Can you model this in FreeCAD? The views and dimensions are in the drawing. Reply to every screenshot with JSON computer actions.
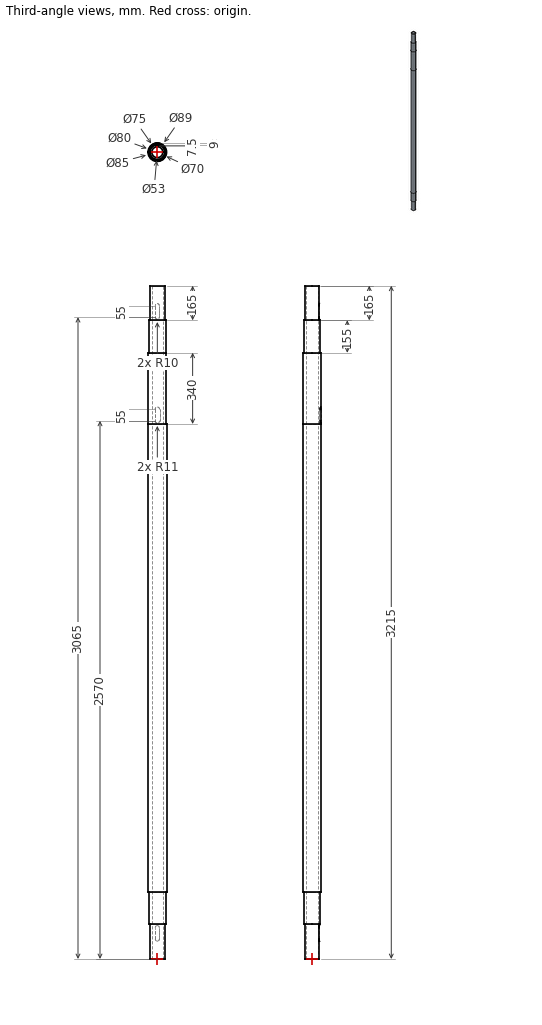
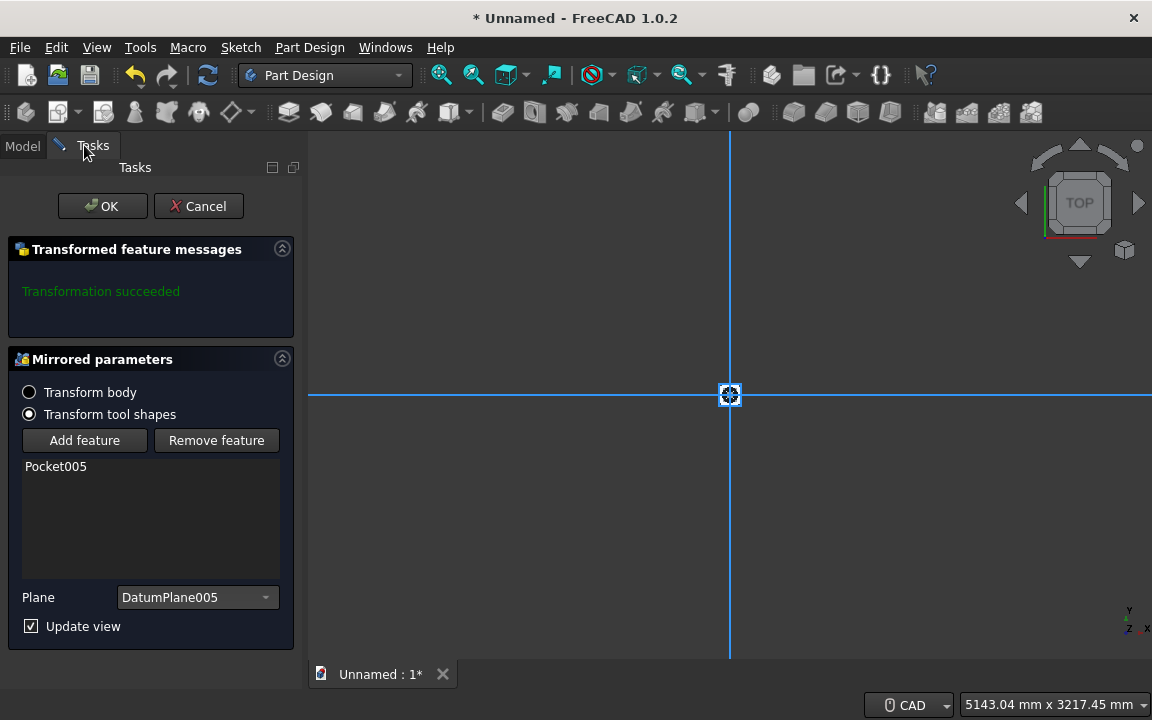
{"action": "left_click", "coordinate": [103, 206]}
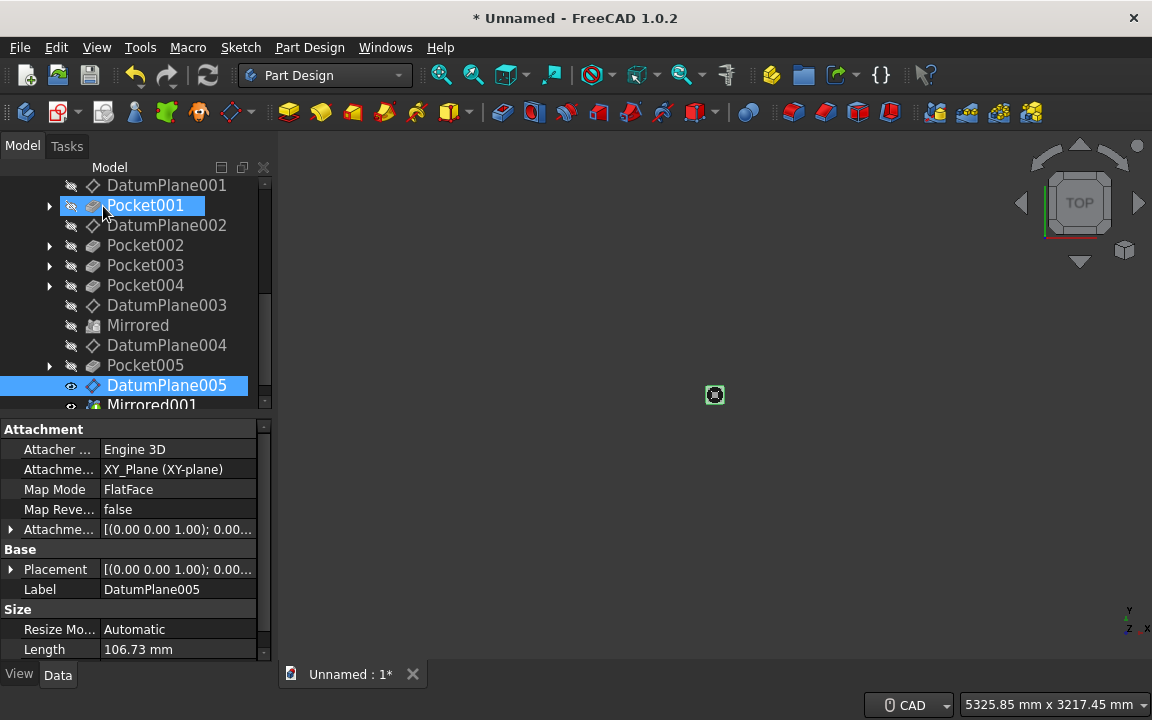
{"action": "left_click", "coordinate": [116, 386]}
{"action": "key", "text": "space"}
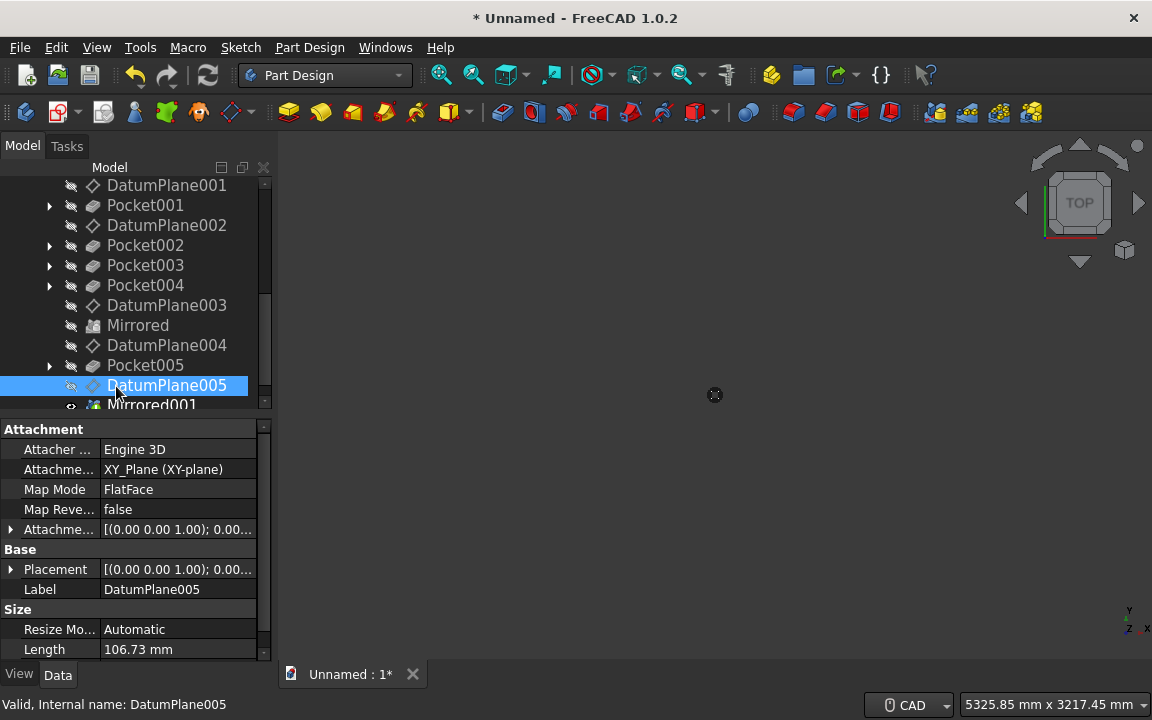
{"action": "left_click", "coordinate": [442, 76]}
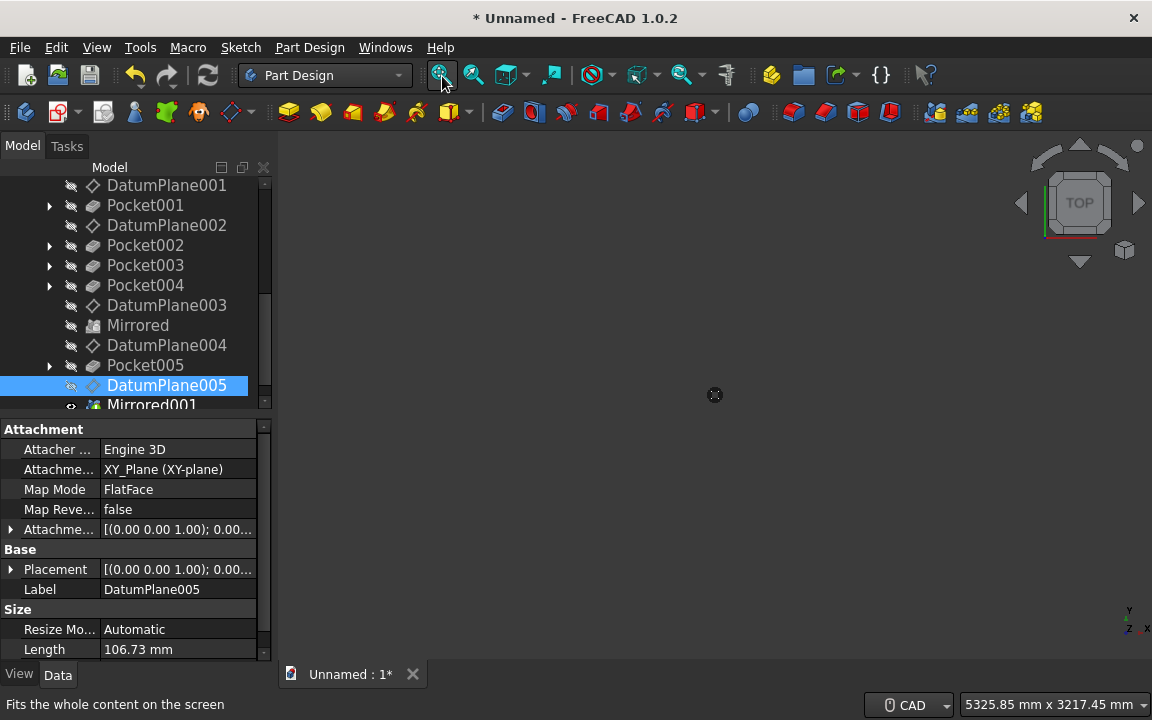
{"action": "scroll", "coordinate": [140, 301], "scroll_direction": "down", "scroll_amount": 3}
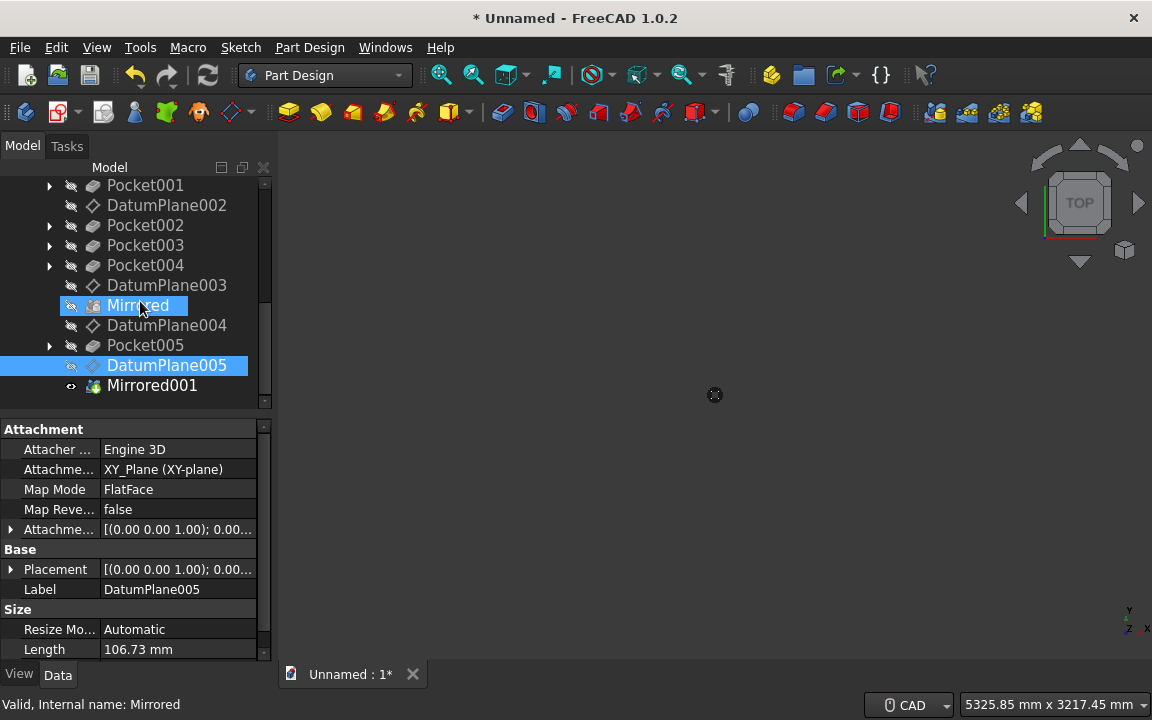
{"action": "scroll", "coordinate": [140, 281], "scroll_direction": "up", "scroll_amount": 15}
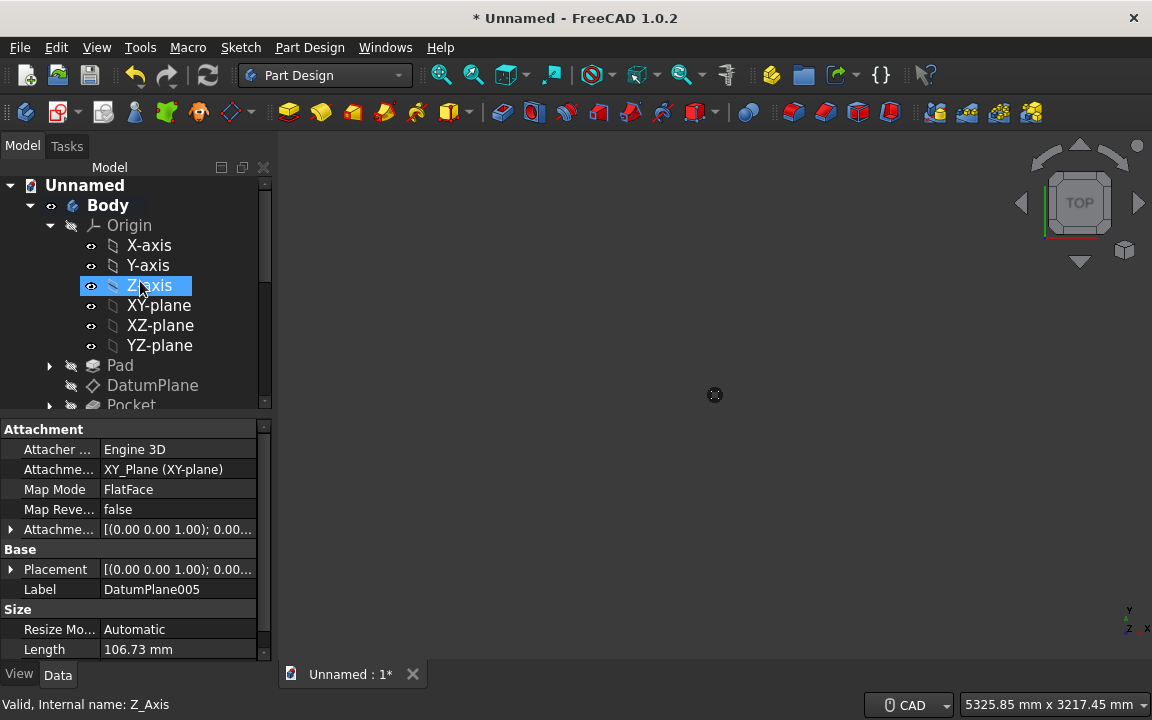
{"action": "left_click", "coordinate": [136, 326]}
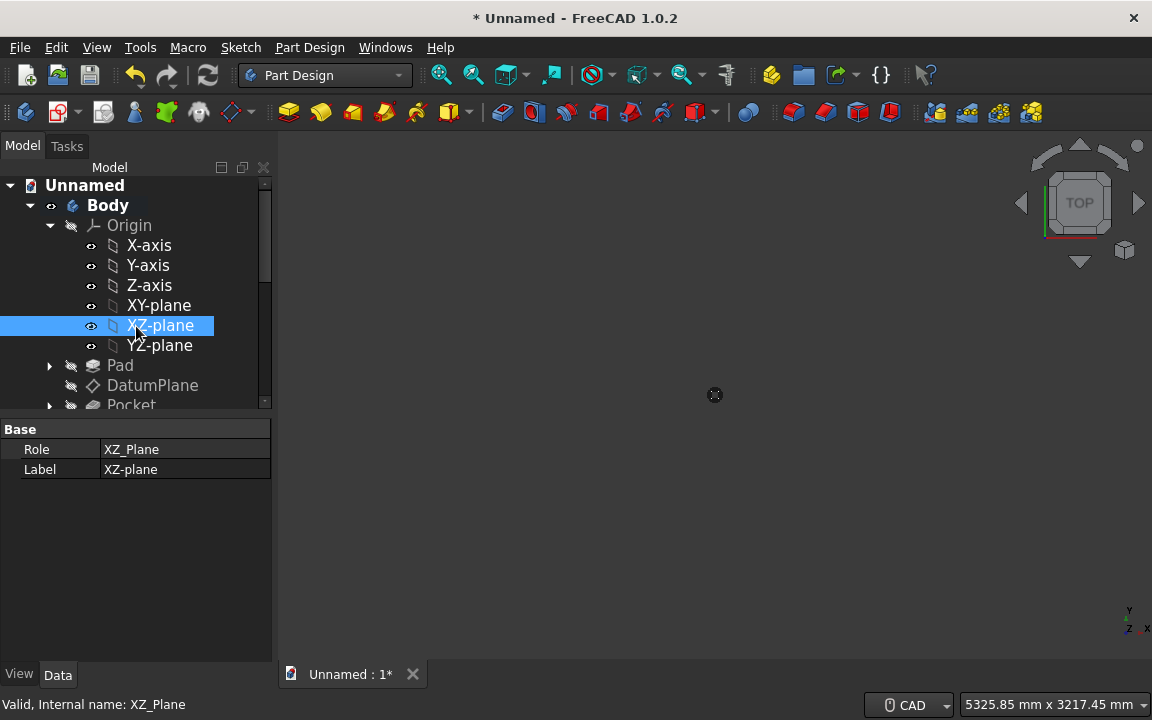
{"action": "left_click", "coordinate": [232, 112]}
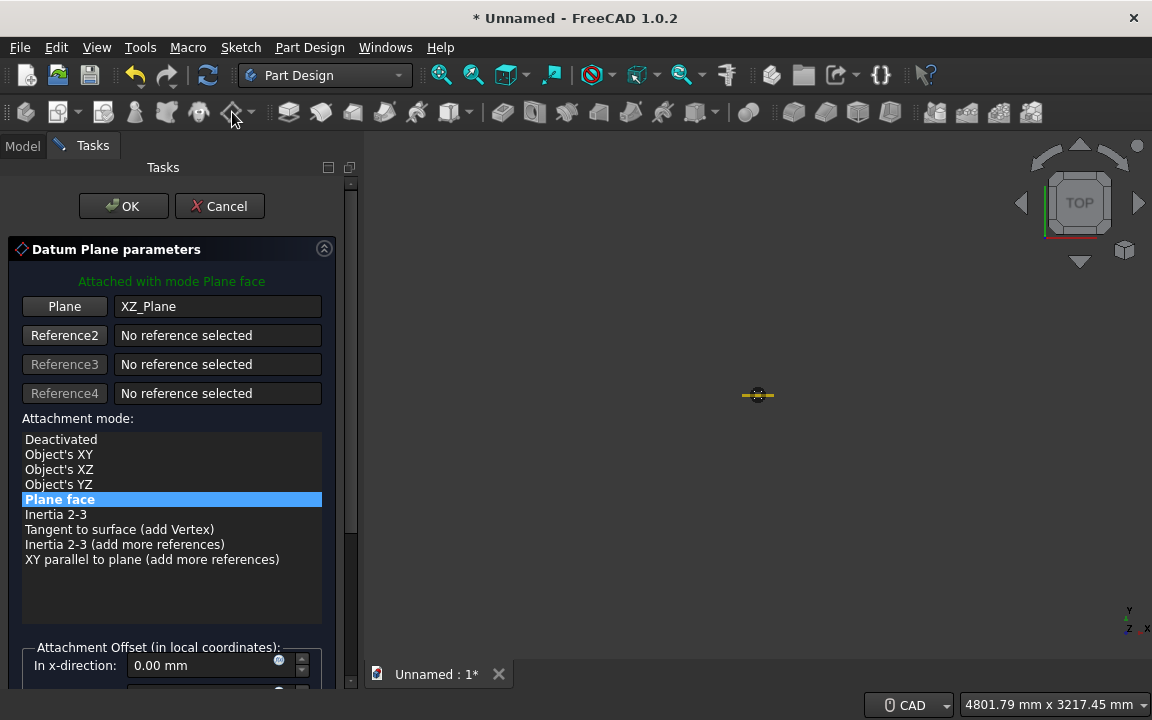
{"action": "scroll", "coordinate": [351, 432], "scroll_direction": "down", "scroll_amount": 2}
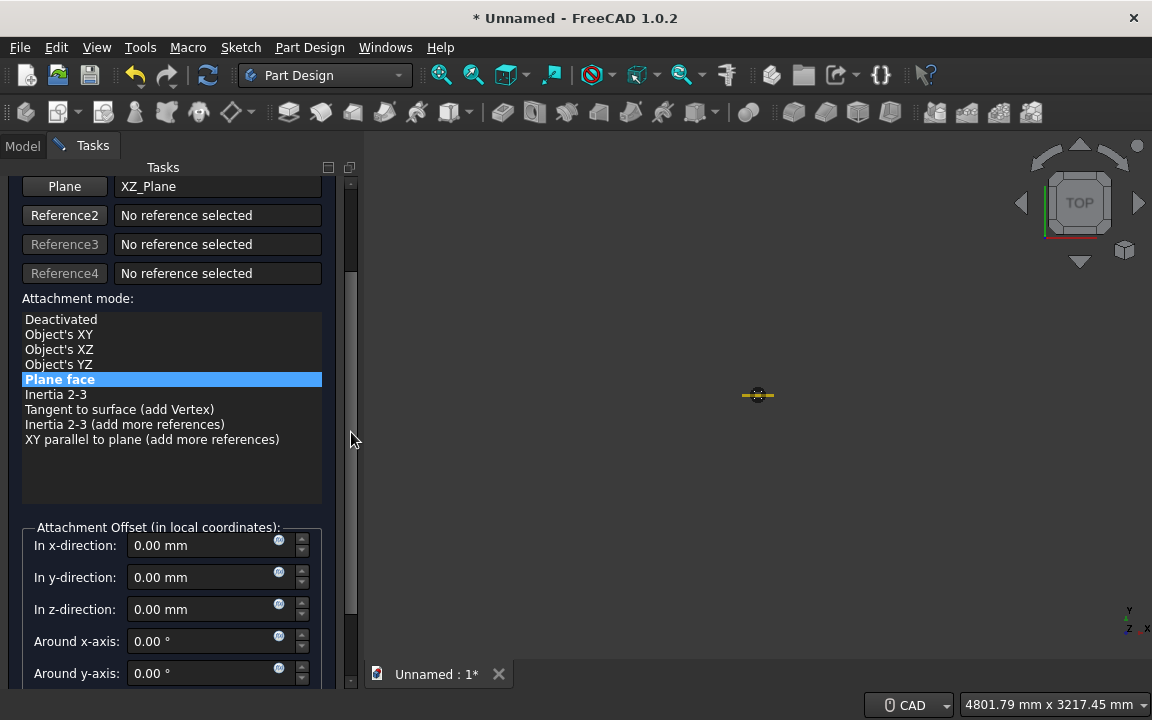
{"action": "triple_click", "coordinate": [210, 609]}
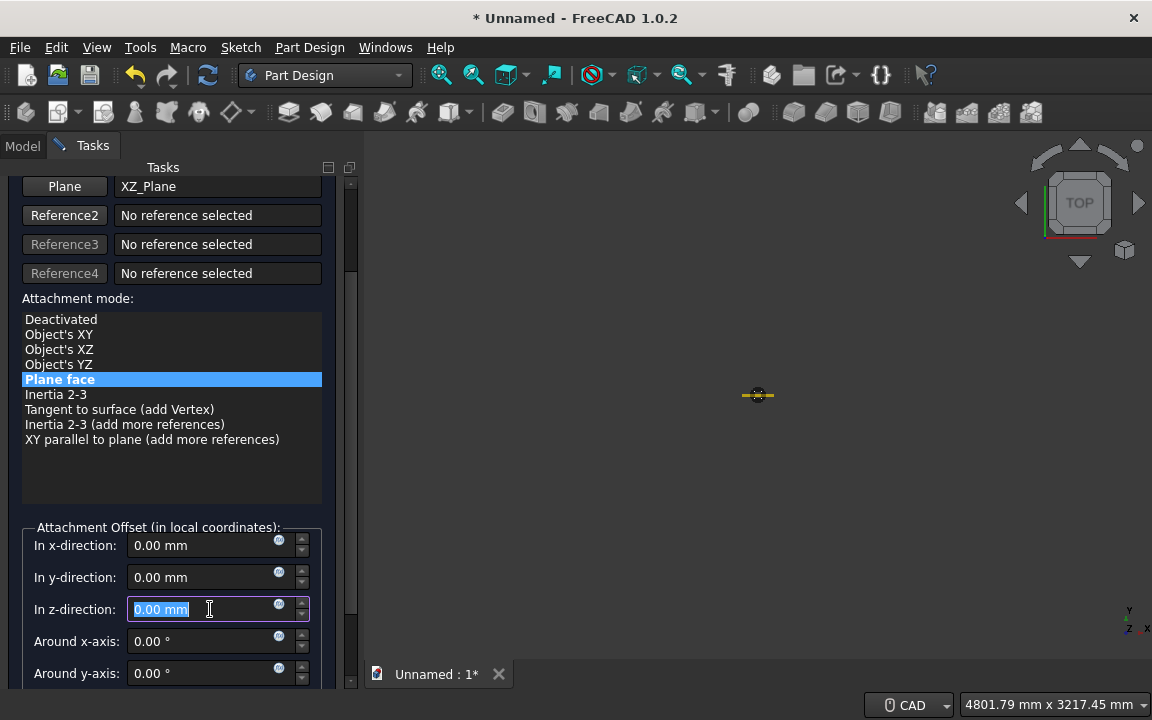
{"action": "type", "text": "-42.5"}
{"action": "key", "text": "Tab"}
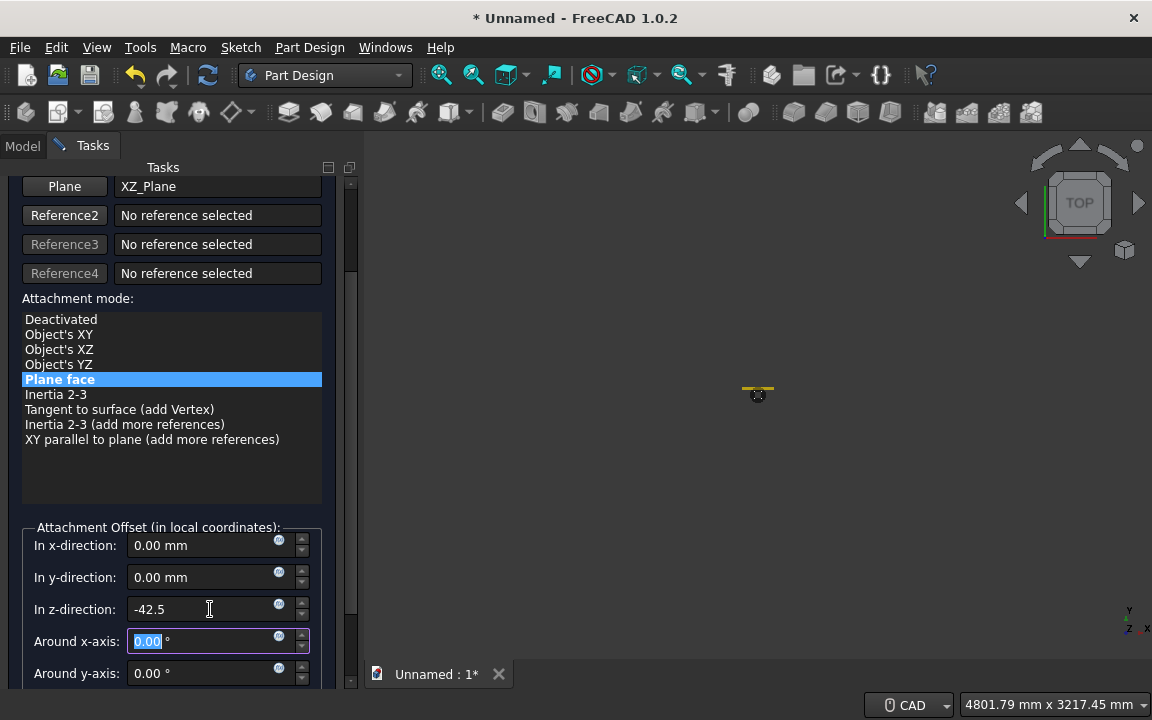
{"action": "scroll", "coordinate": [351, 432], "scroll_direction": "up", "scroll_amount": 3}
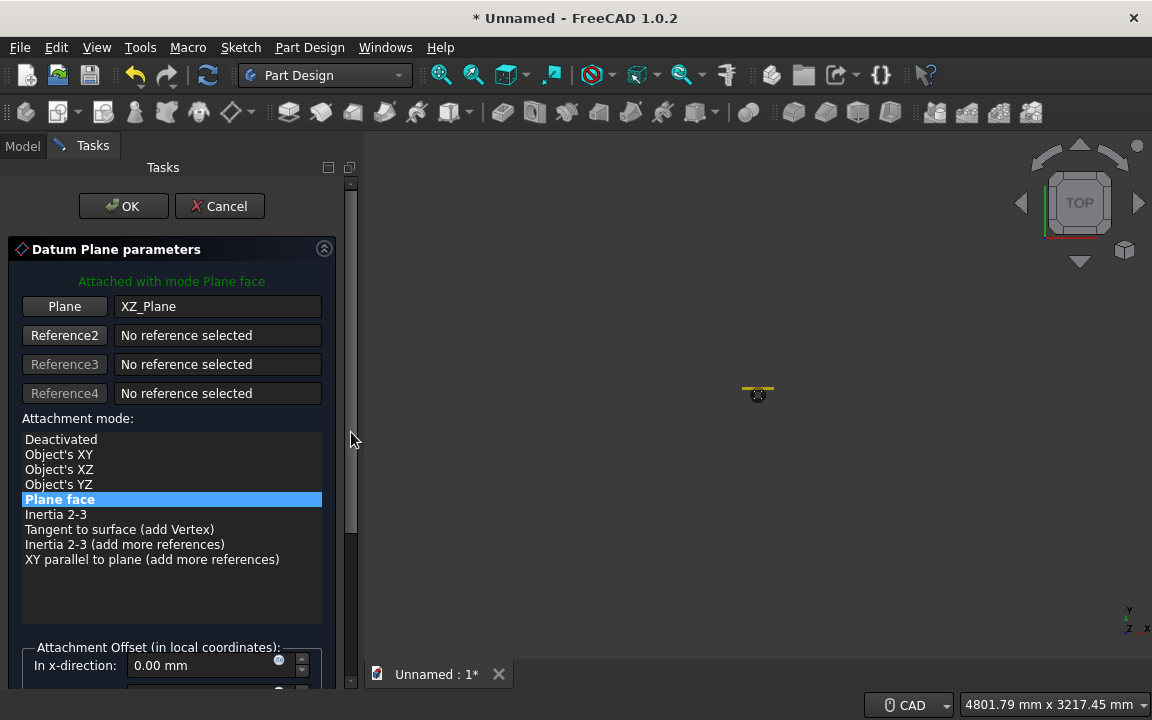
{"action": "left_click", "coordinate": [124, 206]}